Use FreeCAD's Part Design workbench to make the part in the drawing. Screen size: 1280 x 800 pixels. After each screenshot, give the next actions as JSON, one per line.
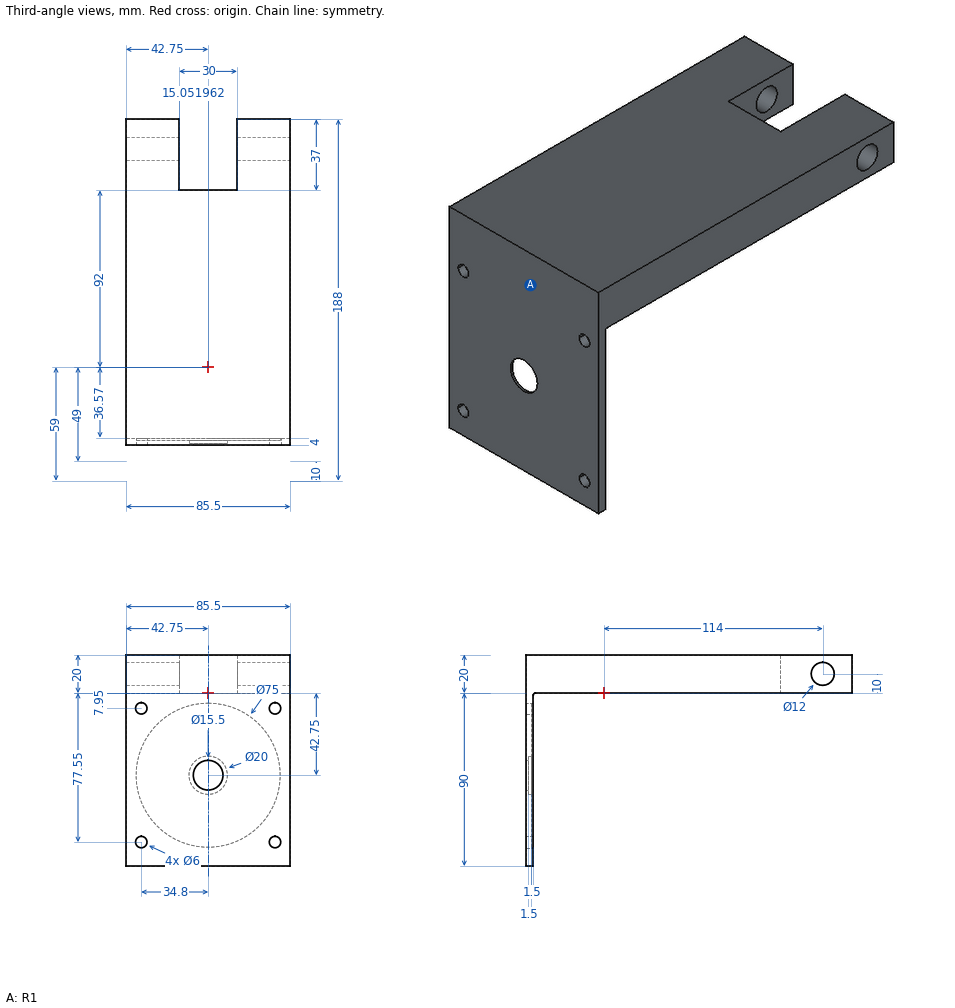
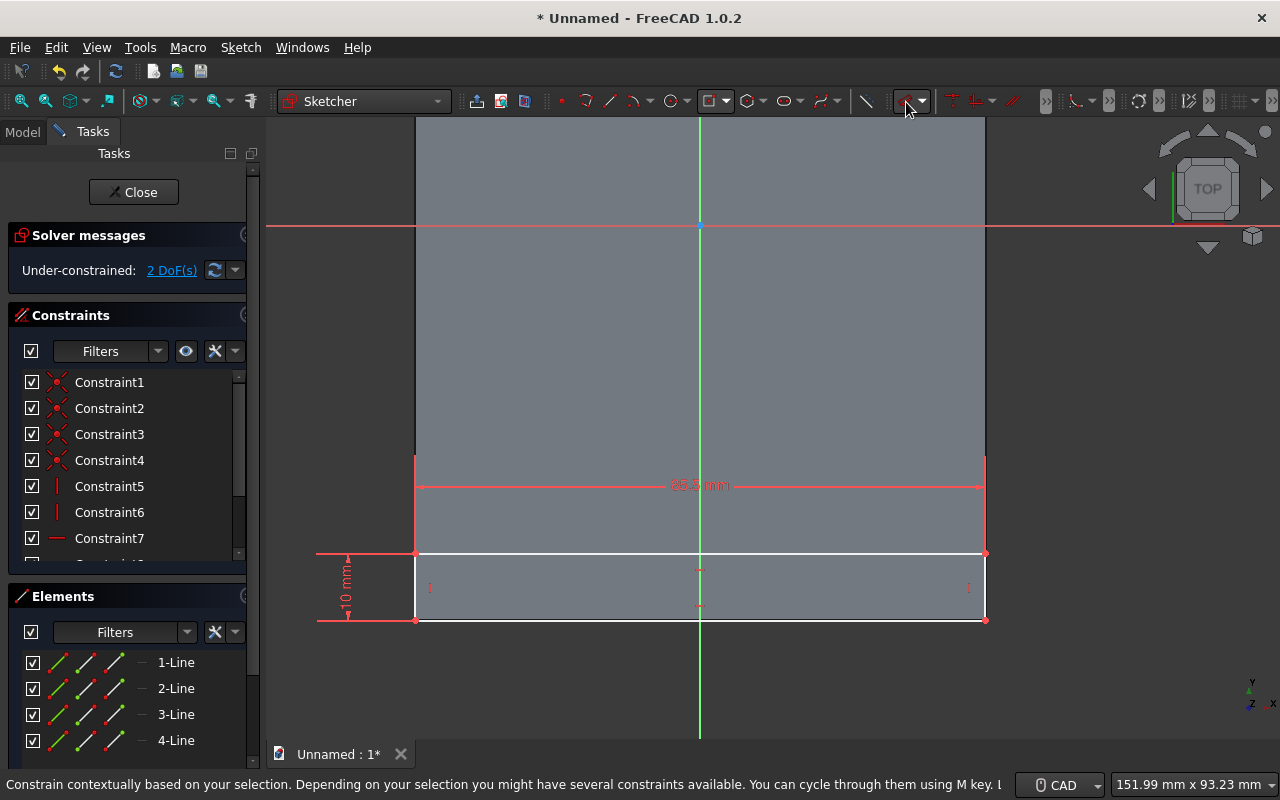
{"action": "left_click", "coordinate": [415, 554]}
{"action": "left_click", "coordinate": [381, 390]}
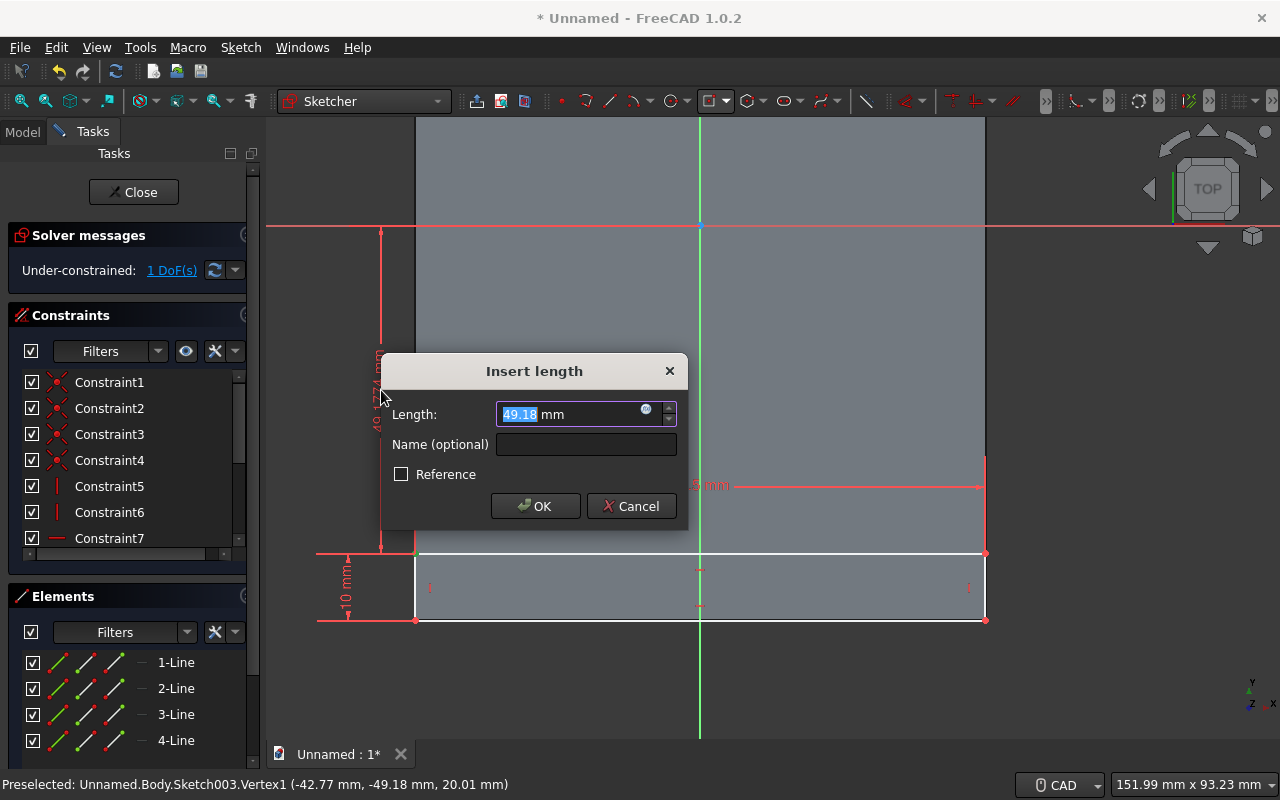
{"action": "type", "text": "49"}
{"action": "key", "text": "Return"}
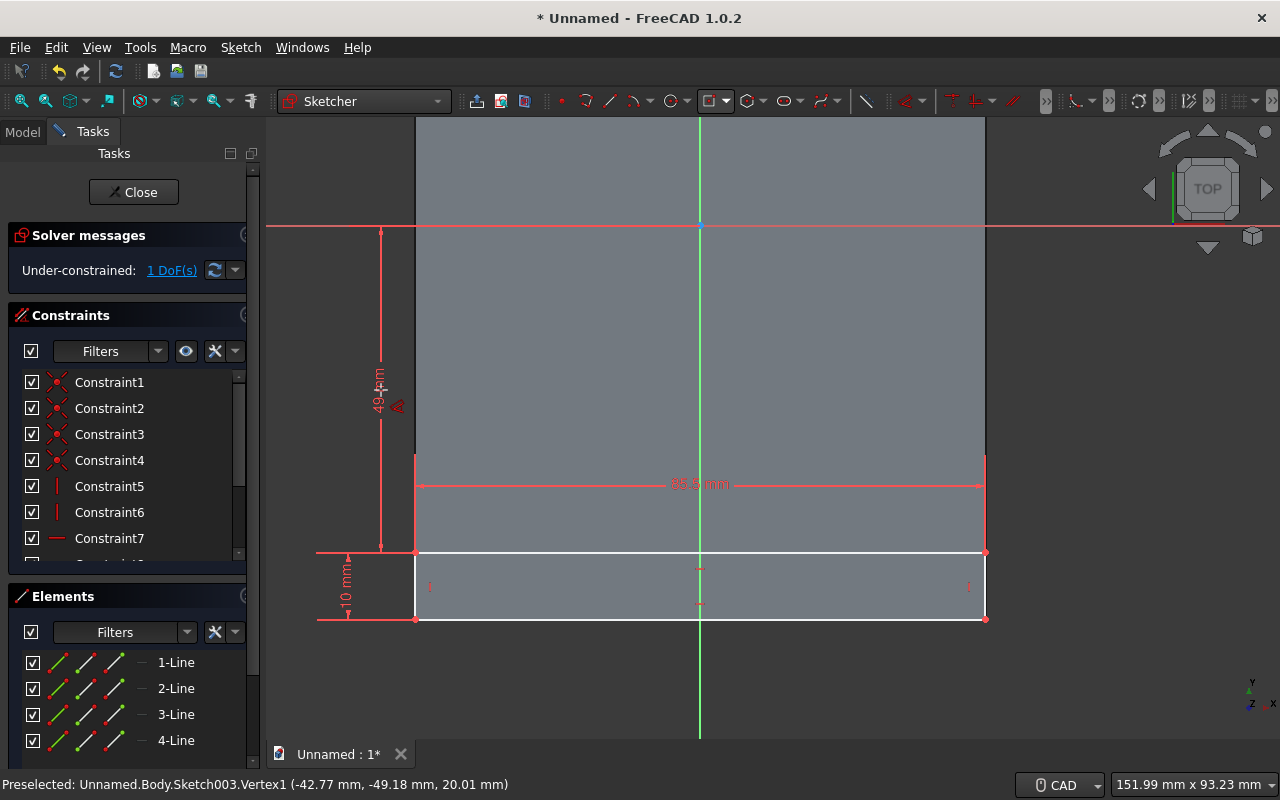
{"action": "left_click", "coordinate": [415, 553]}
{"action": "left_click", "coordinate": [558, 192]}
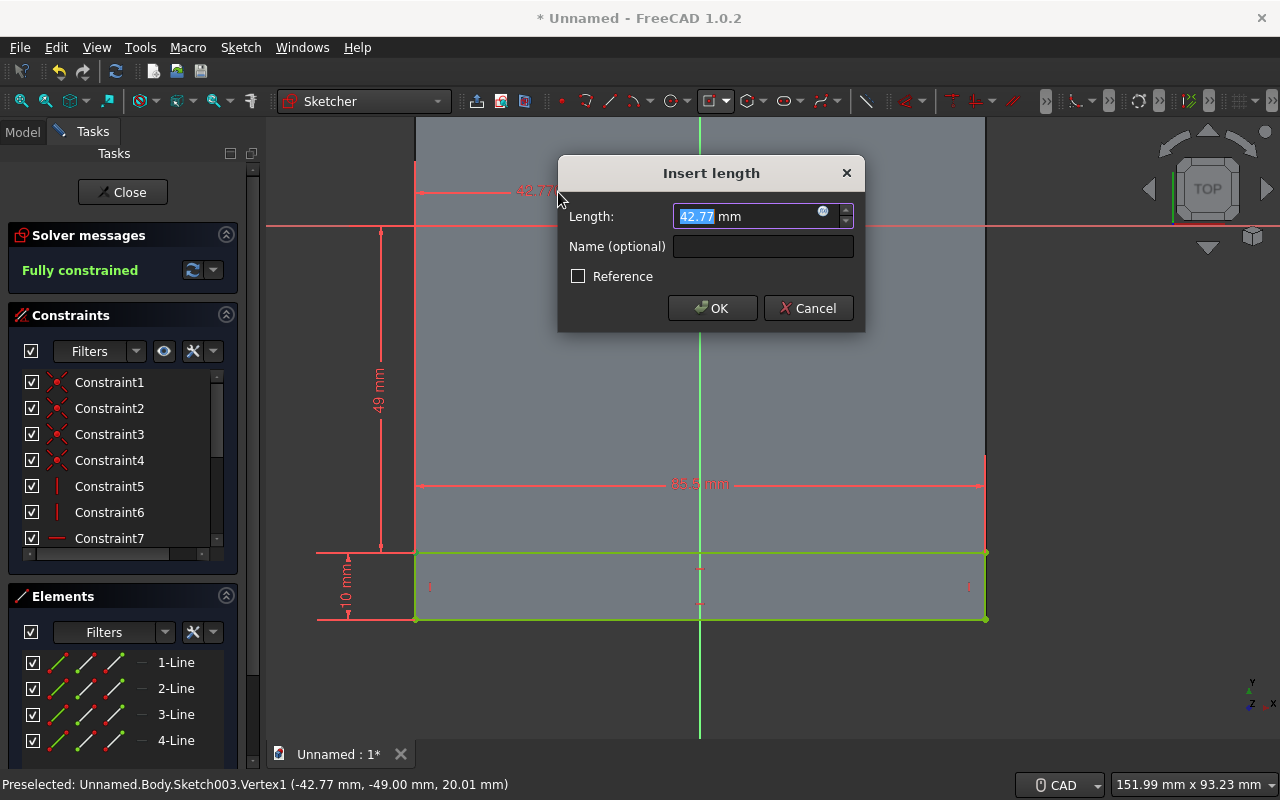
{"action": "type", "text": "42.75"}
{"action": "key", "text": "Return"}
{"action": "key", "text": "Escape"}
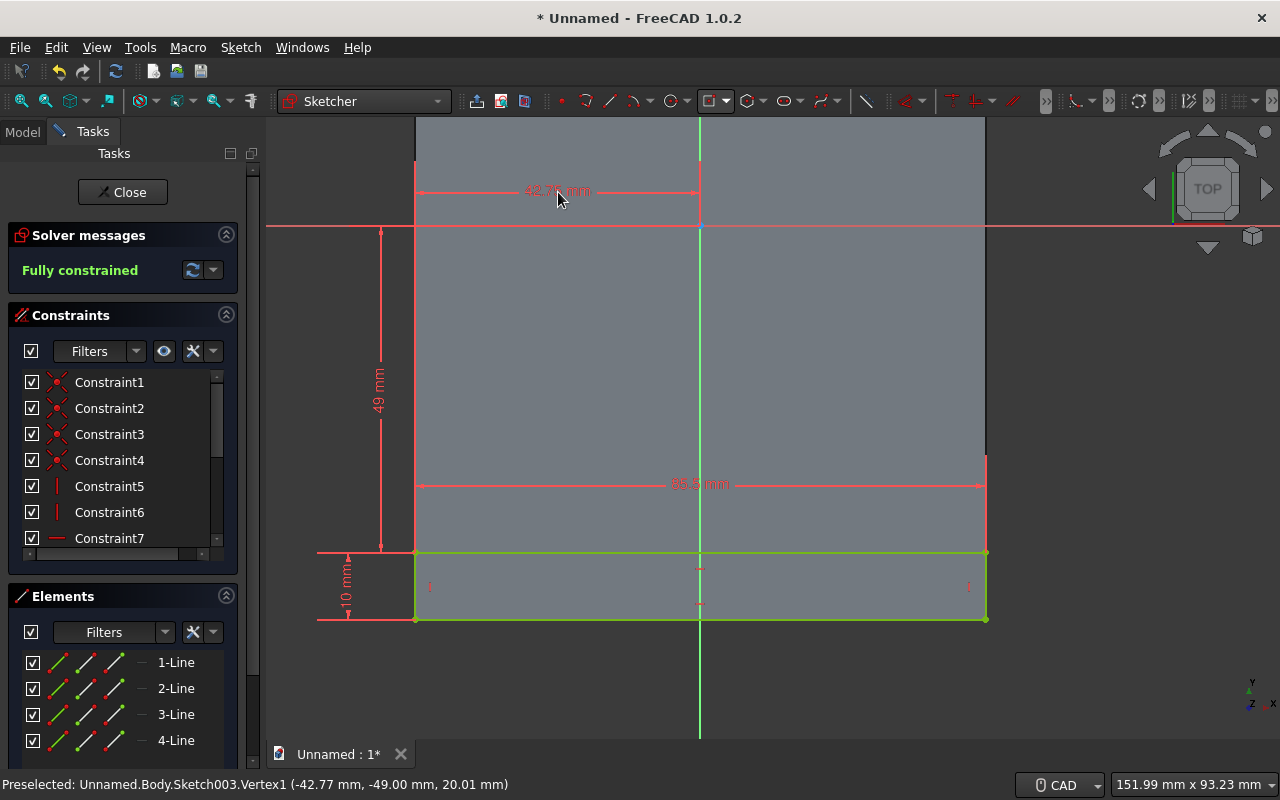
{"action": "left_click", "coordinate": [123, 192]}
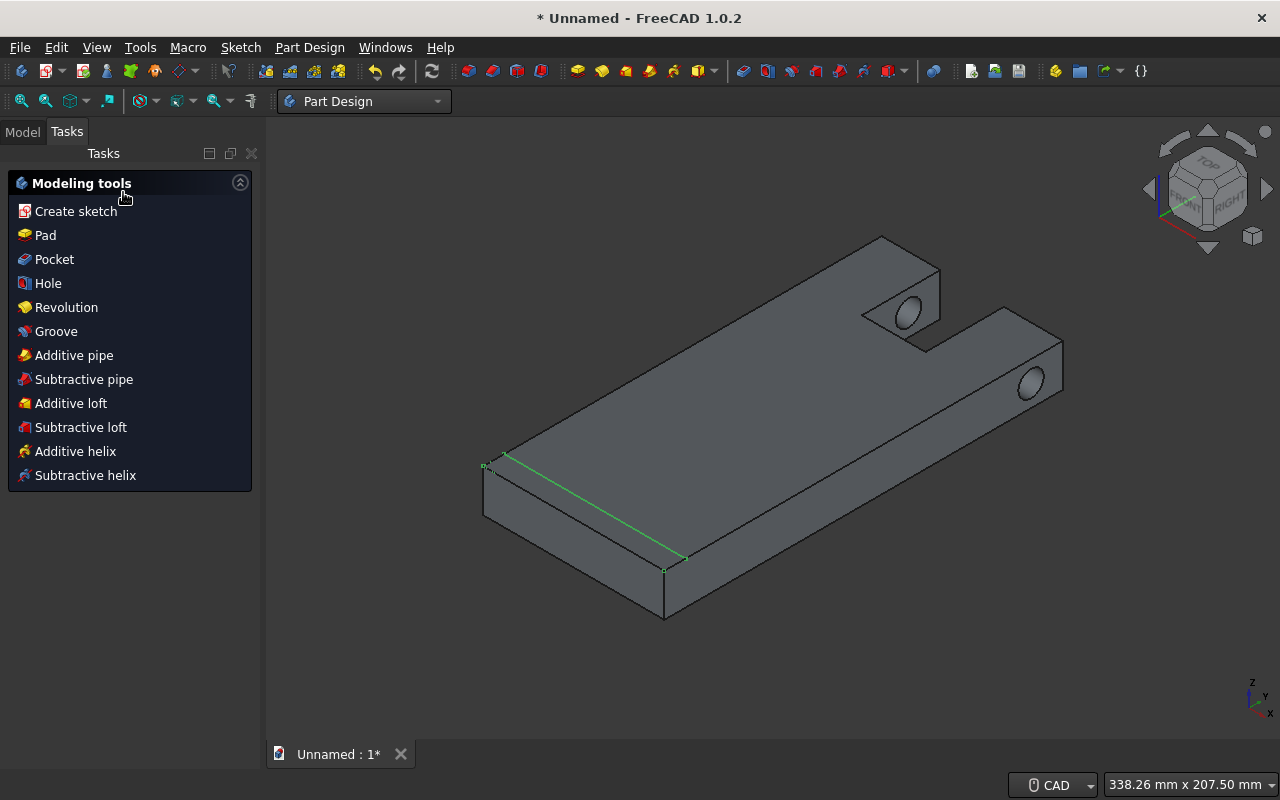
{"action": "left_click", "coordinate": [744, 72]}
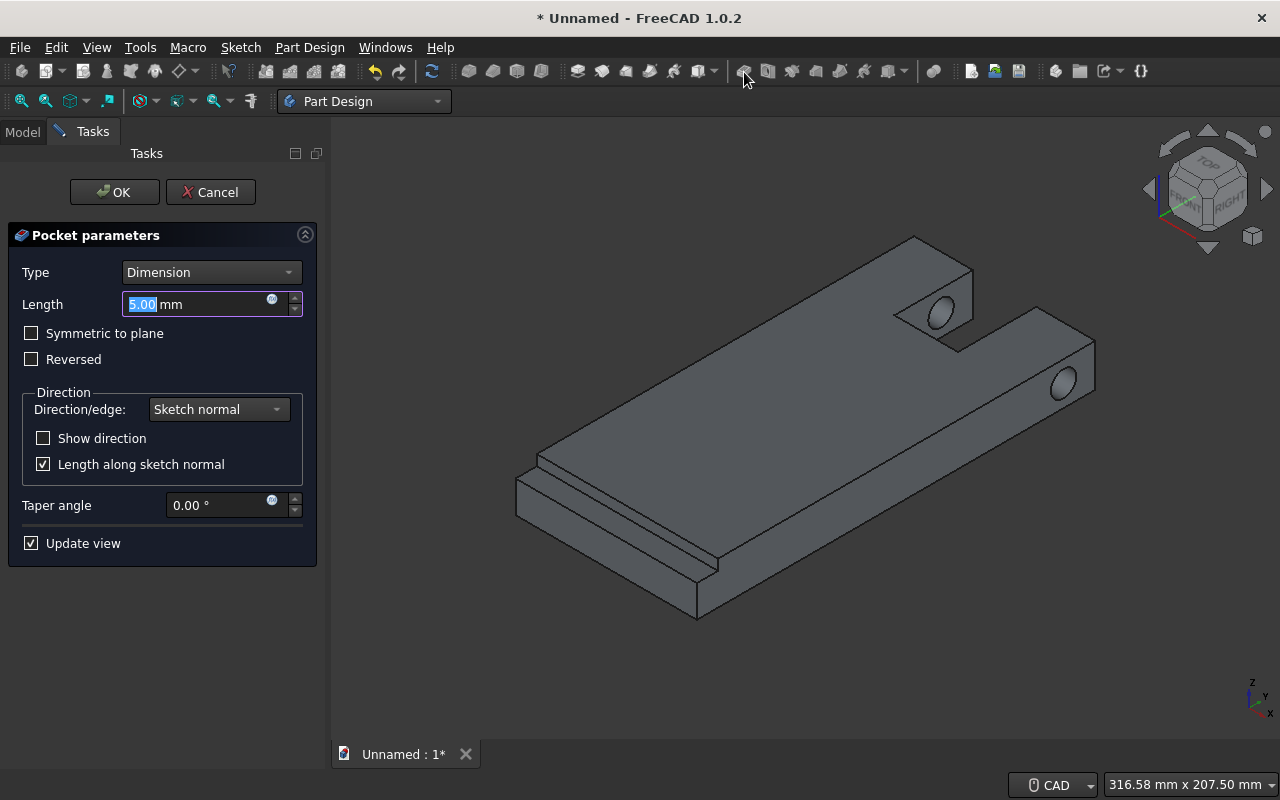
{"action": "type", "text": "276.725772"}
{"action": "key", "text": "Tab"}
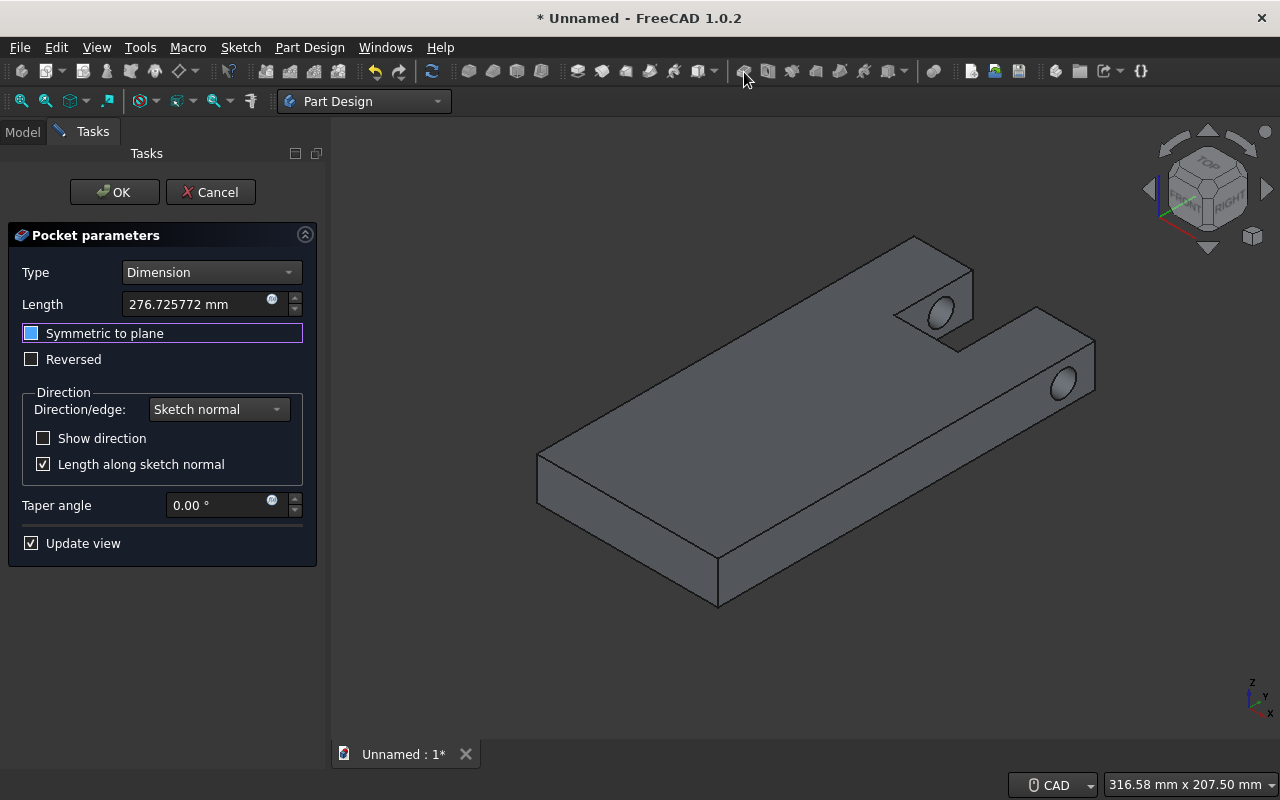
{"action": "left_click", "coordinate": [30, 333]}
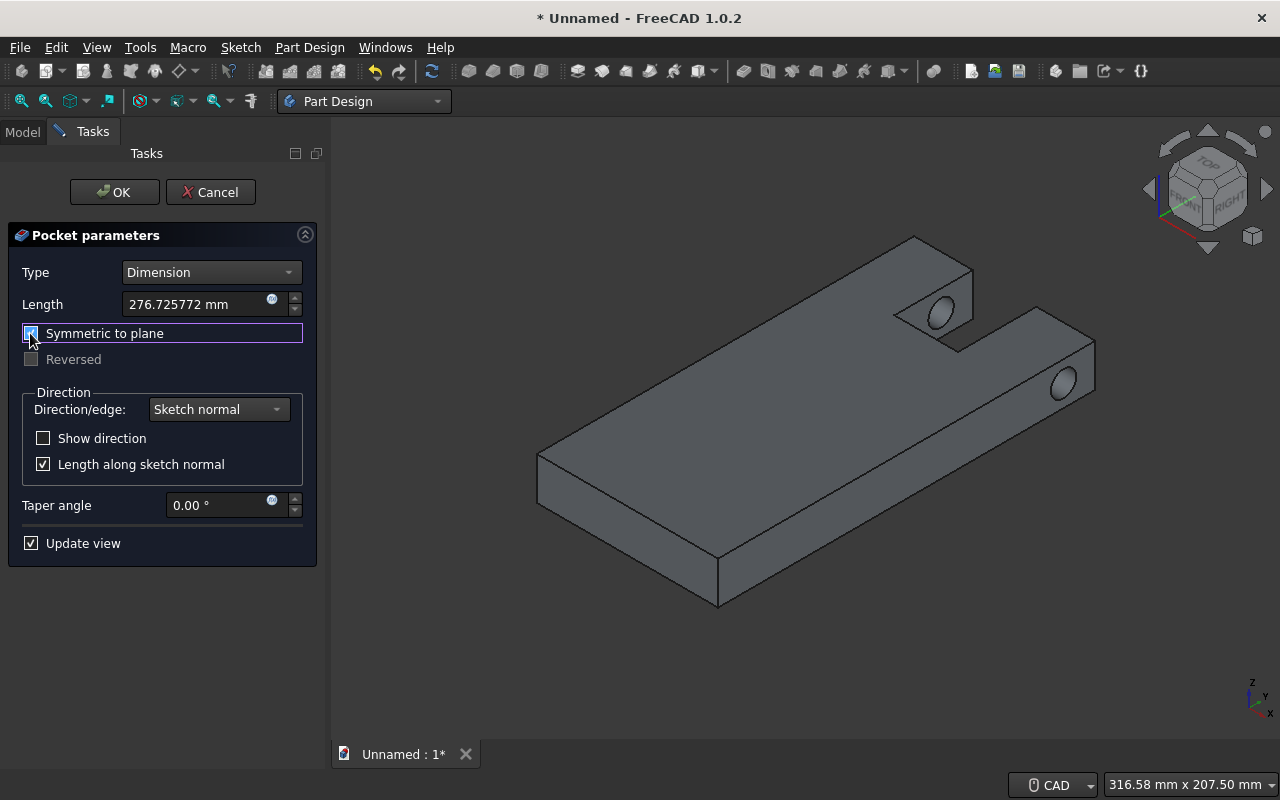
{"action": "left_click", "coordinate": [115, 192]}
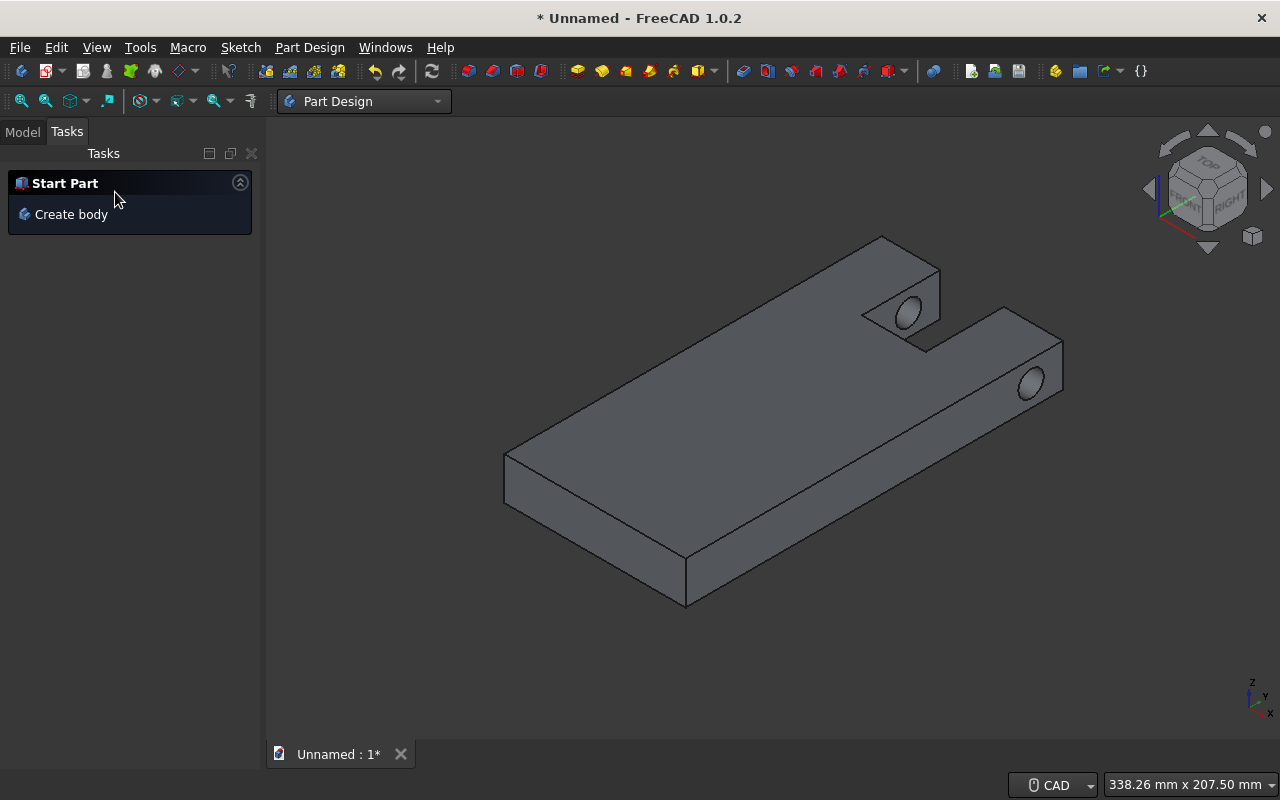
{"action": "left_click", "coordinate": [647, 560]}